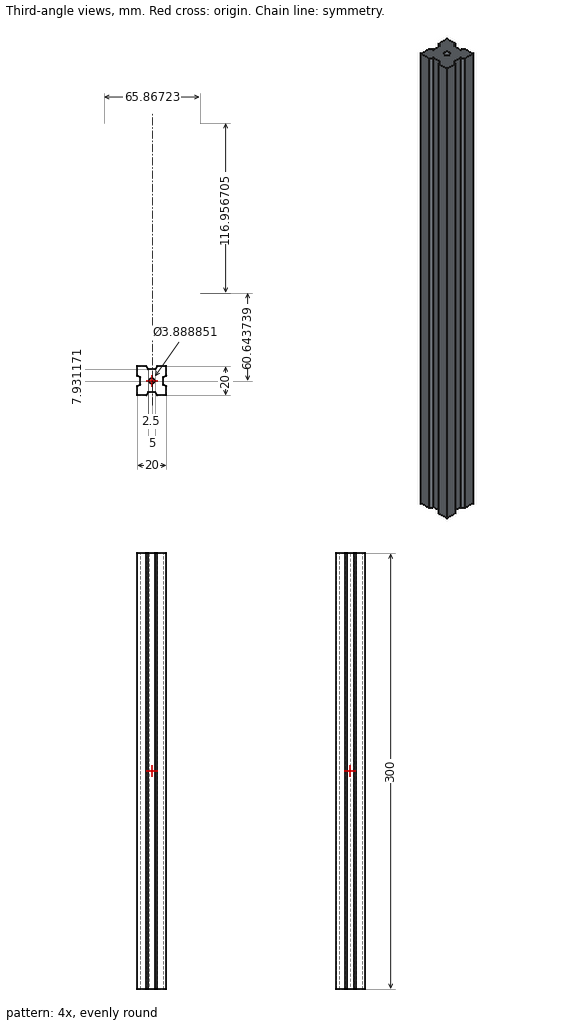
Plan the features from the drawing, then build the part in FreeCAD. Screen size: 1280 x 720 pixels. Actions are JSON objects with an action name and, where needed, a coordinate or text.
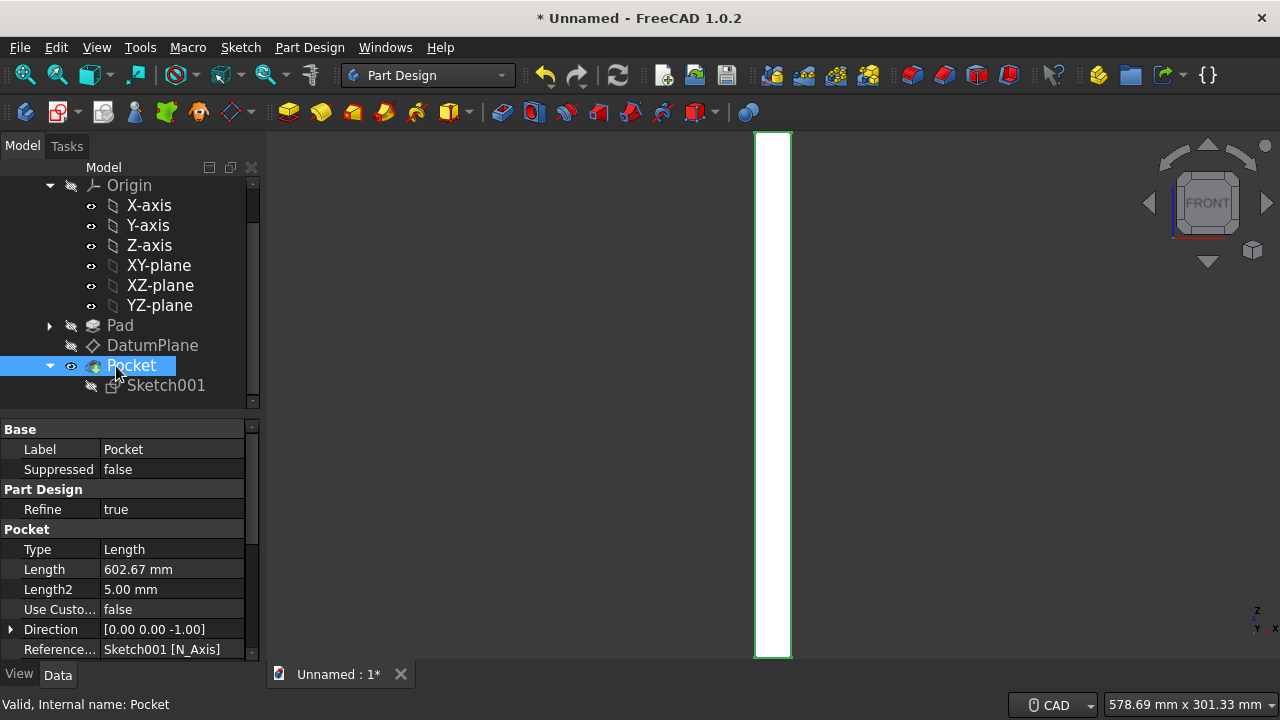
{"action": "left_click", "coordinate": [836, 76]}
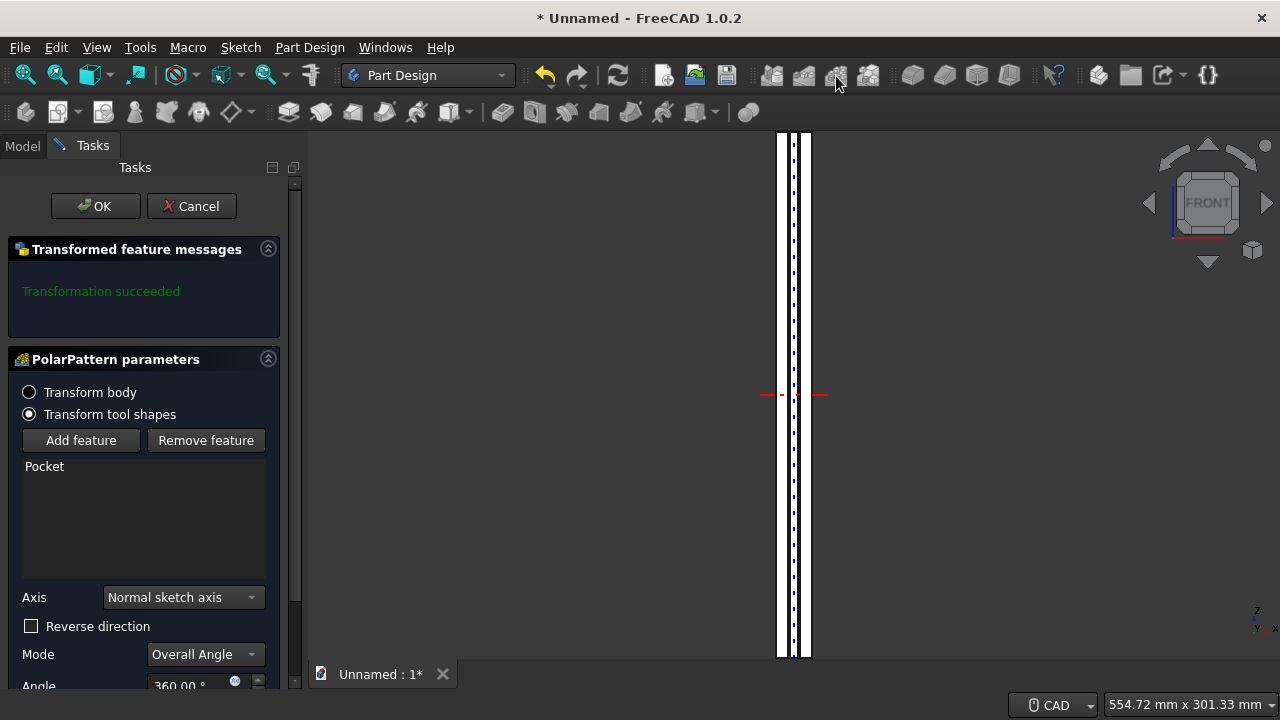
{"action": "left_click", "coordinate": [184, 598]}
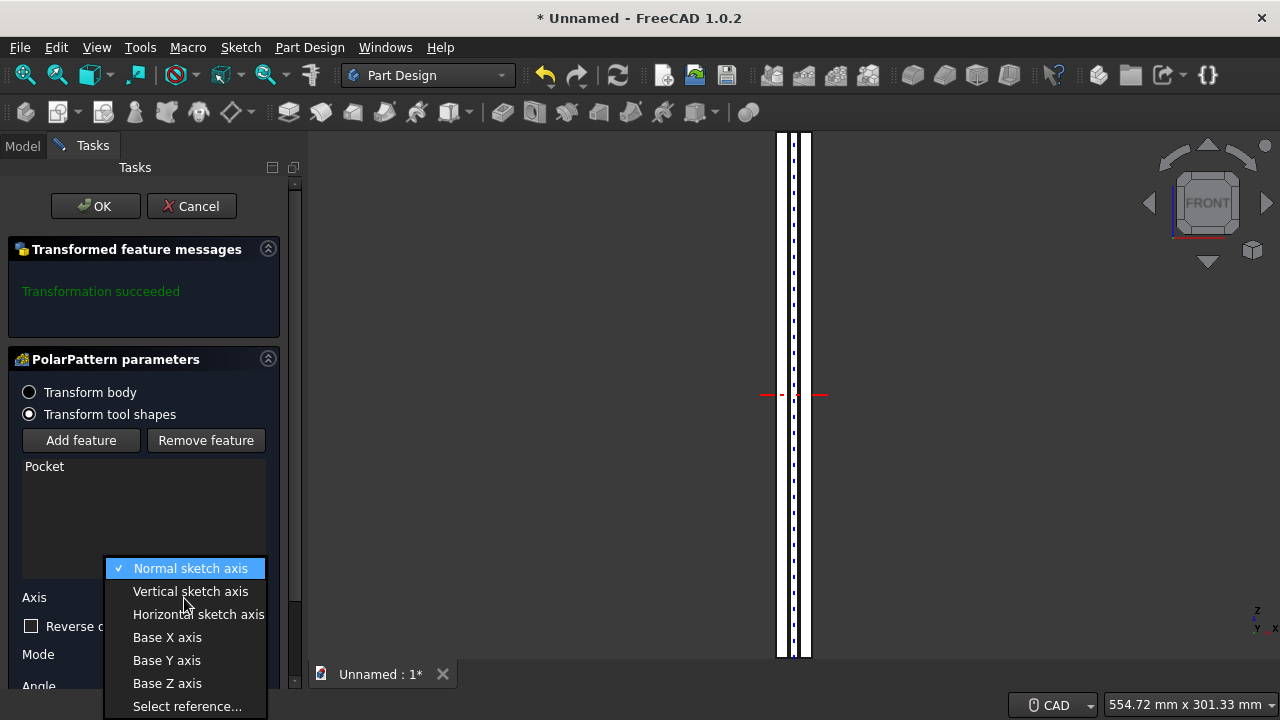
{"action": "left_click", "coordinate": [184, 684]}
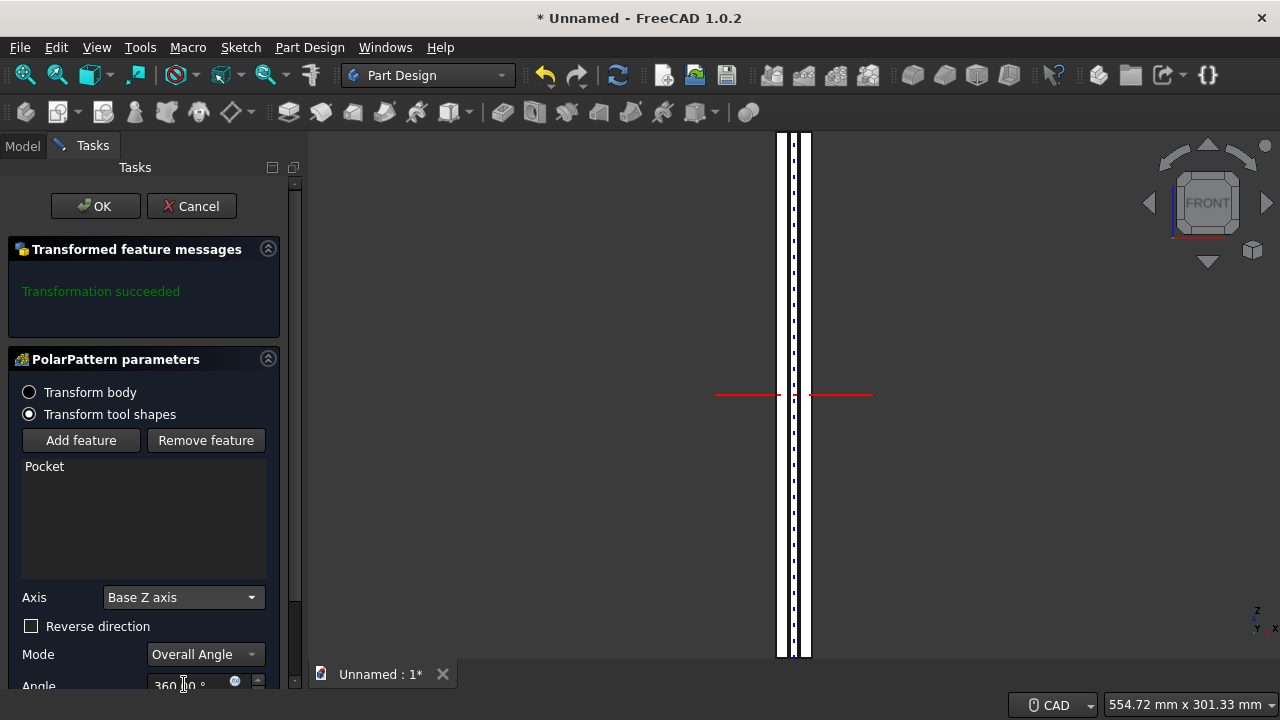
{"action": "scroll", "coordinate": [295, 432], "scroll_direction": "down", "scroll_amount": 2}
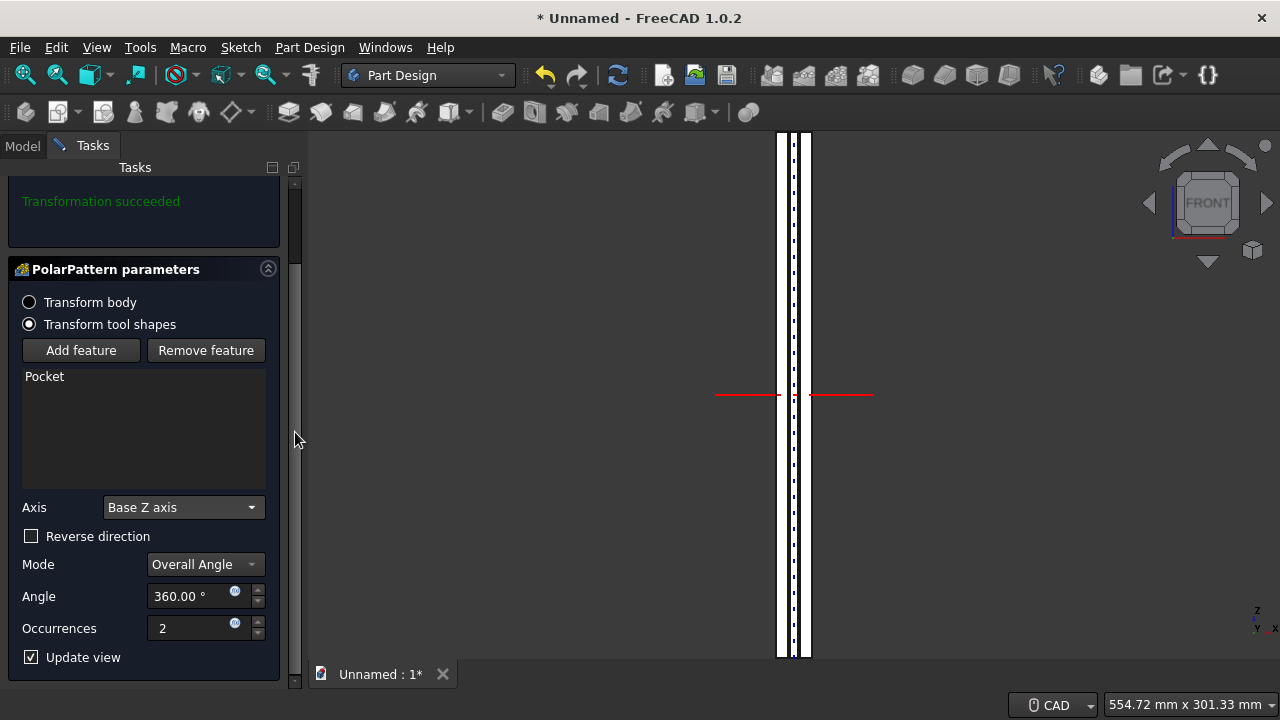
{"action": "triple_click", "coordinate": [198, 628]}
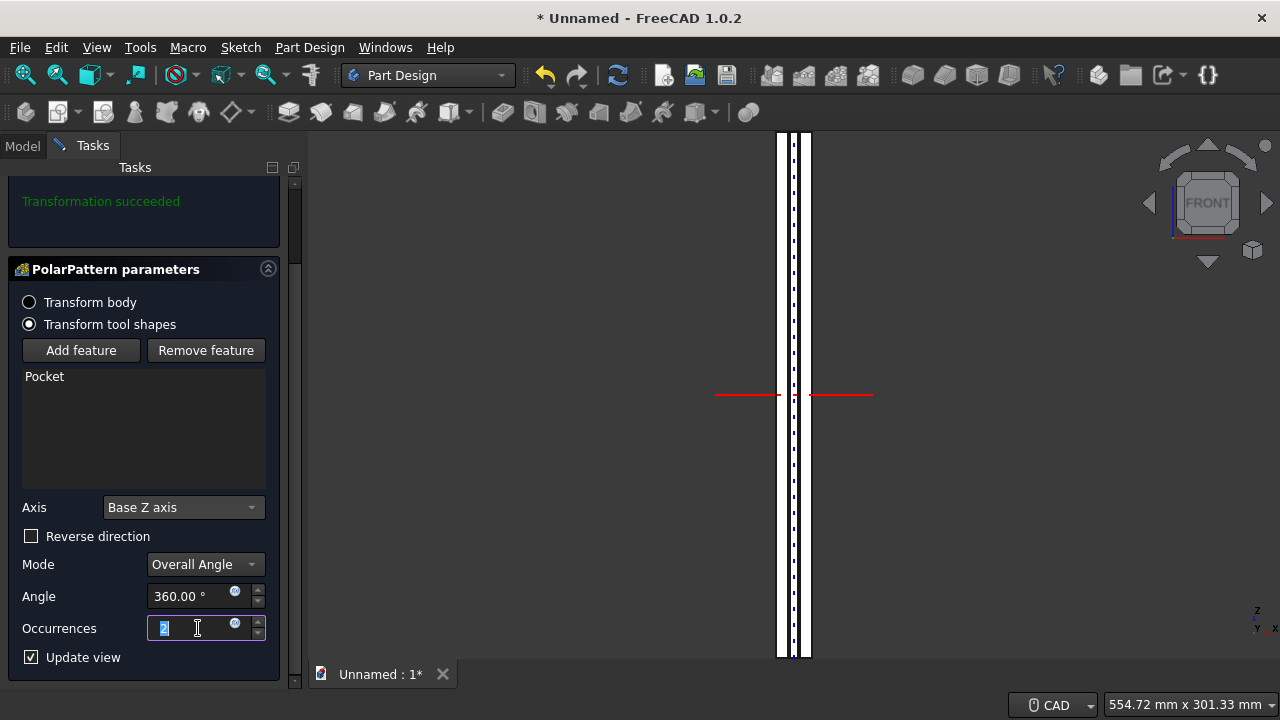
{"action": "type", "text": "4"}
{"action": "key", "text": "Tab"}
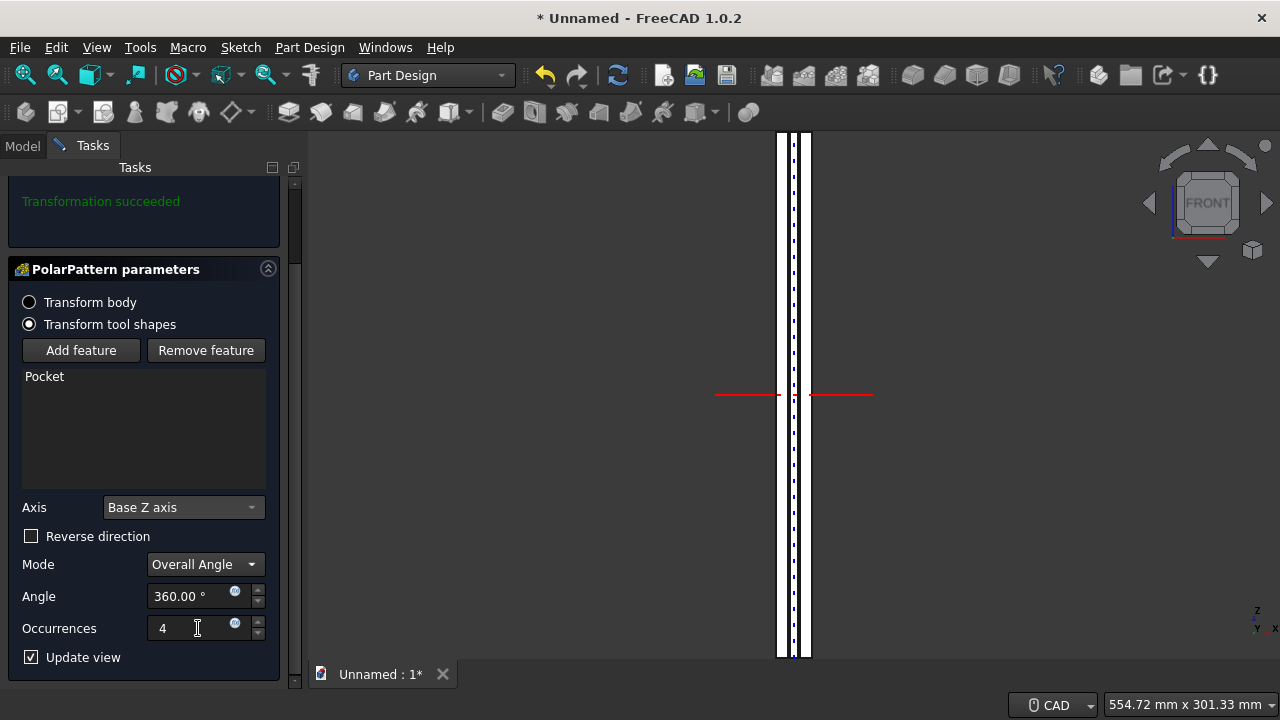
{"action": "scroll", "coordinate": [295, 432], "scroll_direction": "up", "scroll_amount": 3}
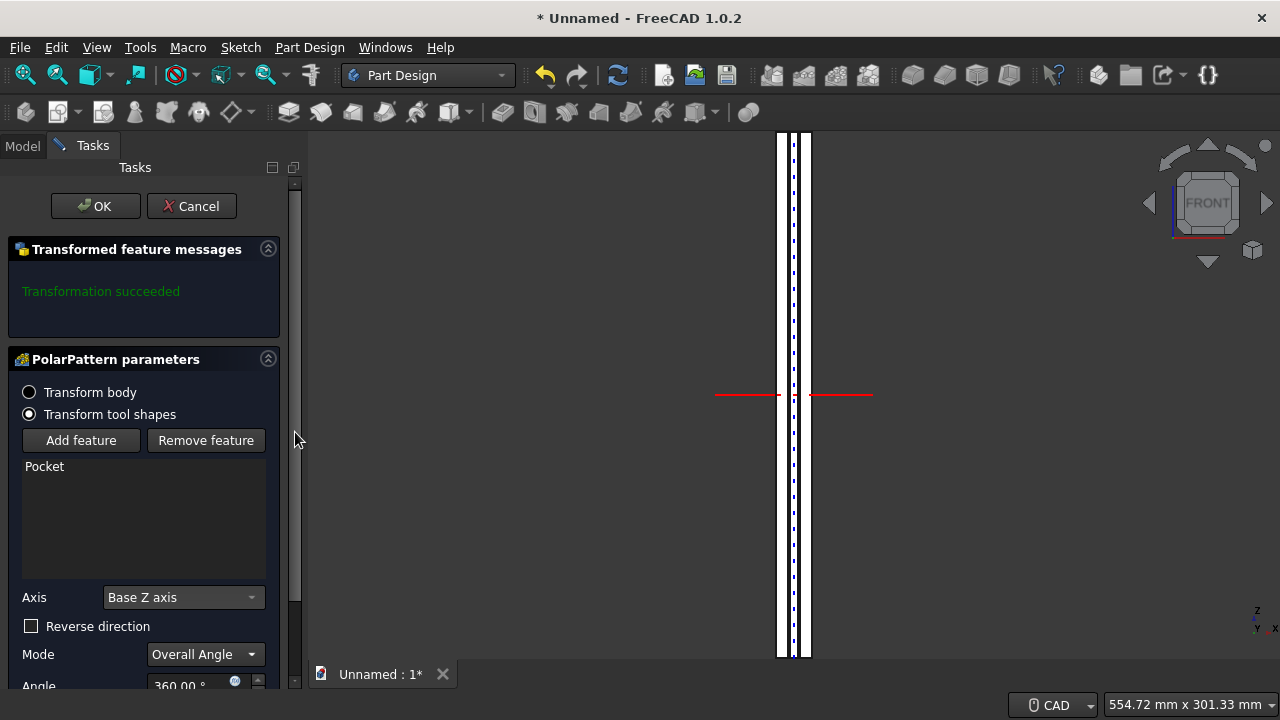
{"action": "left_click", "coordinate": [96, 206]}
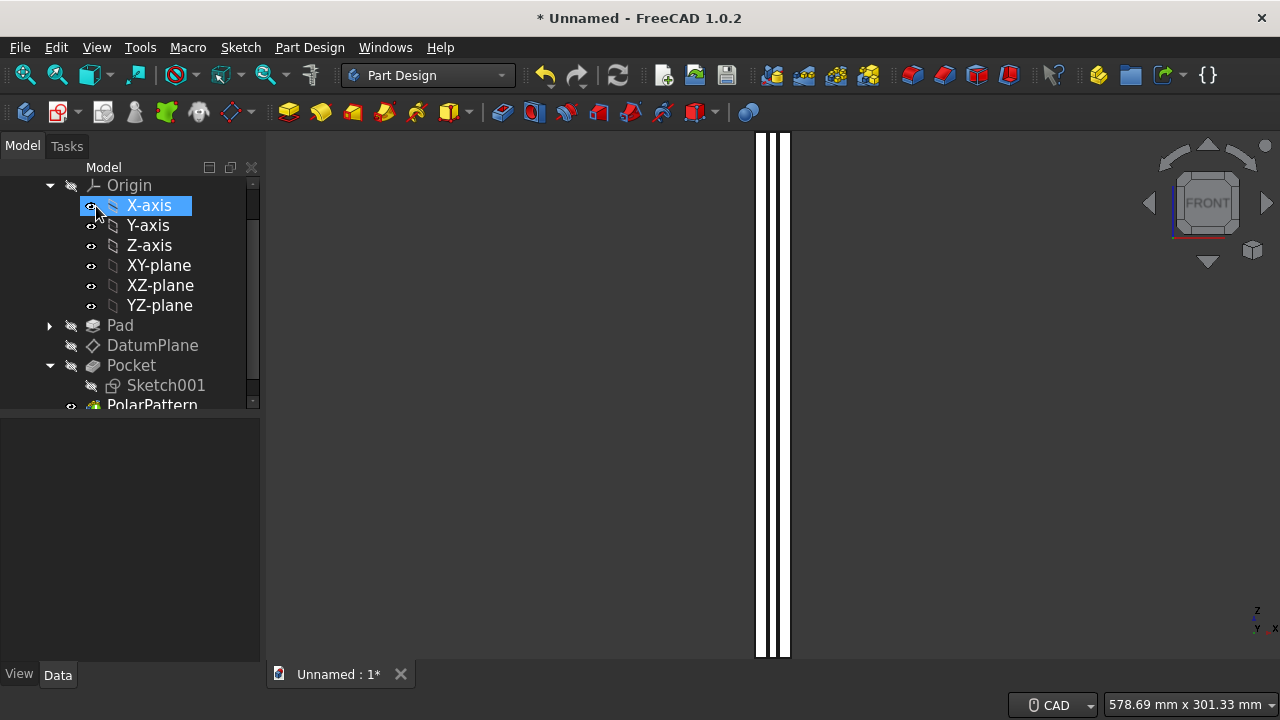
{"action": "key", "text": "0"}